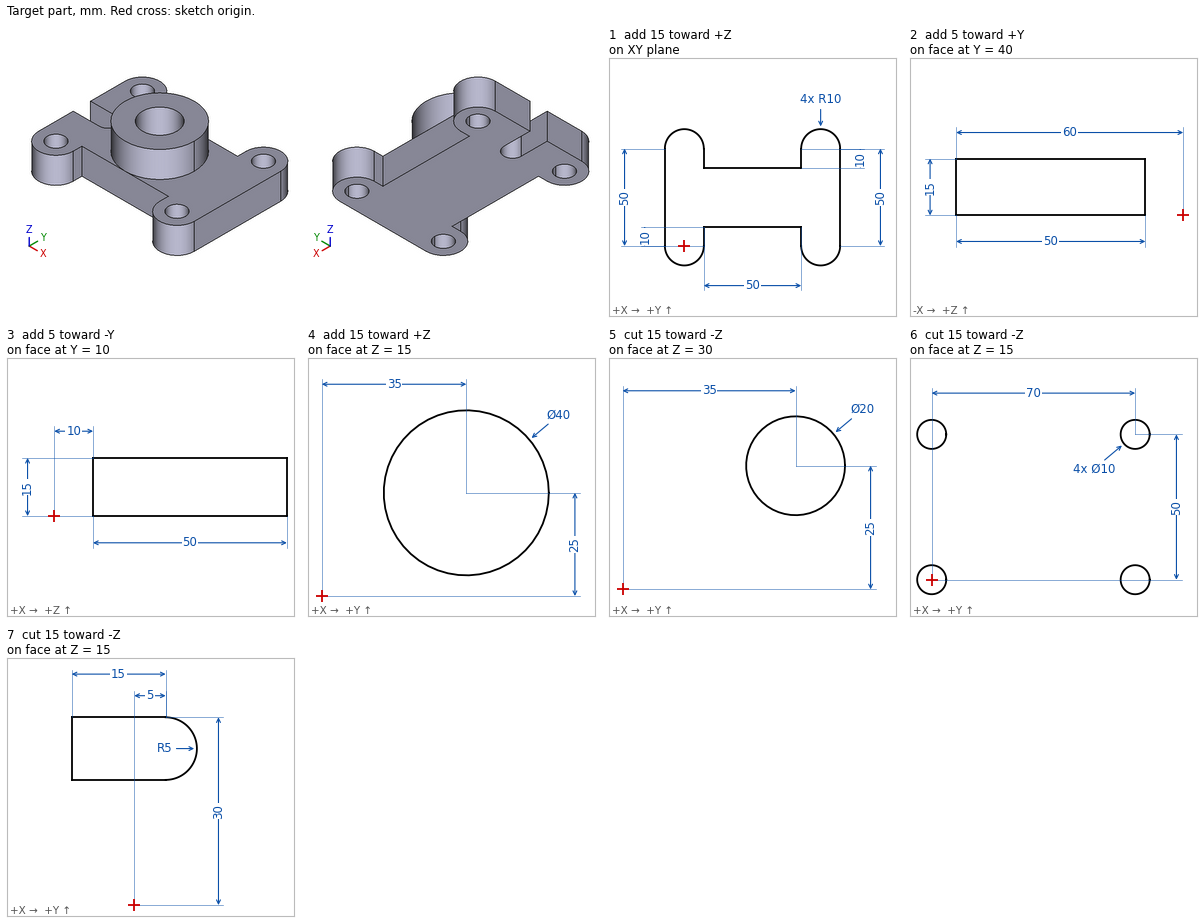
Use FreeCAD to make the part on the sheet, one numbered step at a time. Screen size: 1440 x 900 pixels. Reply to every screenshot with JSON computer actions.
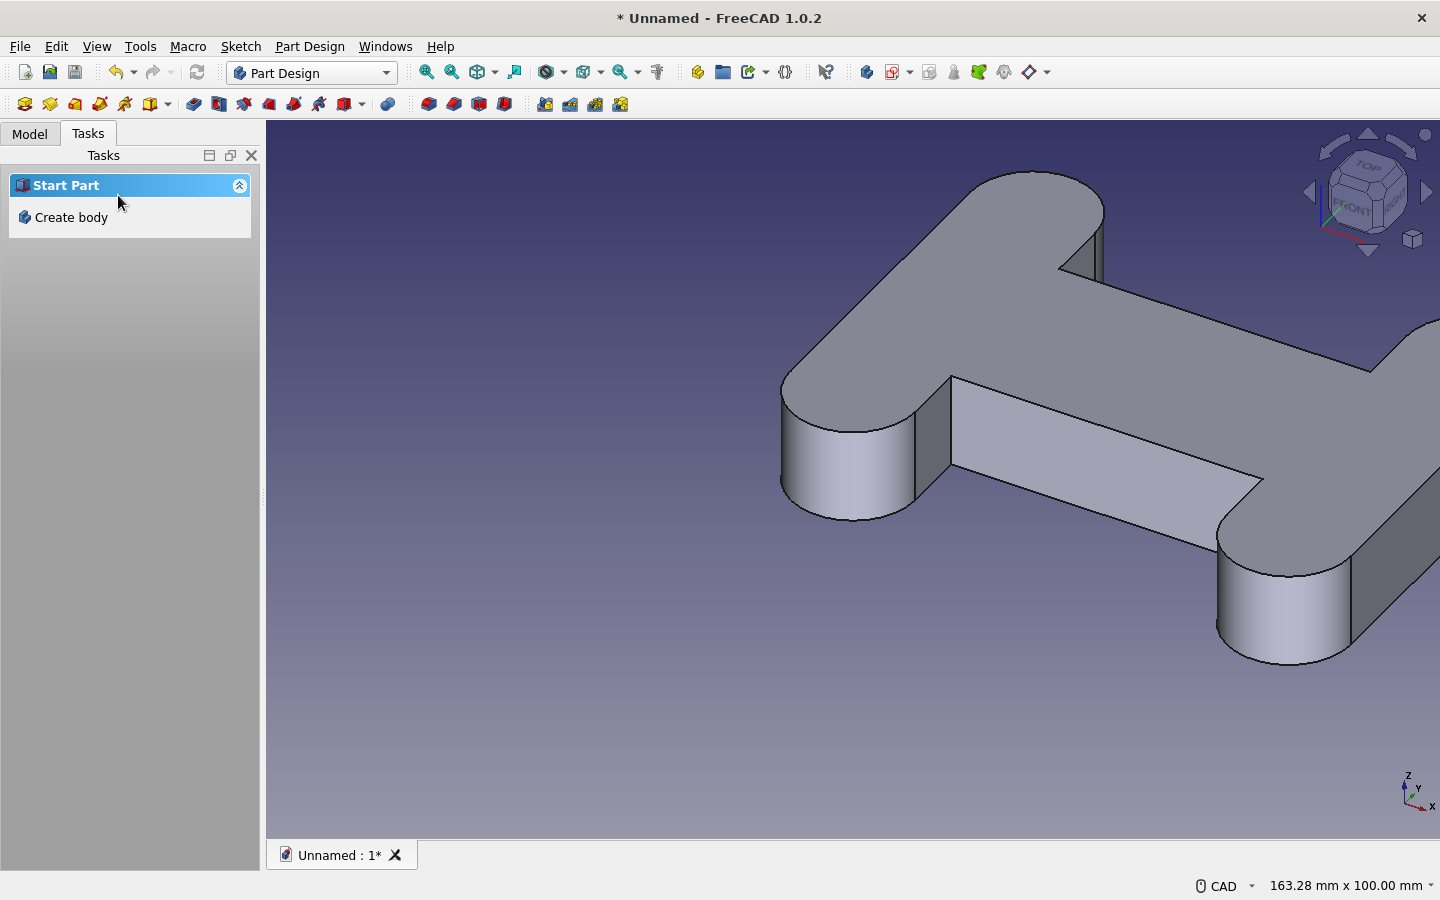
{"action": "left_click", "coordinate": [427, 72]}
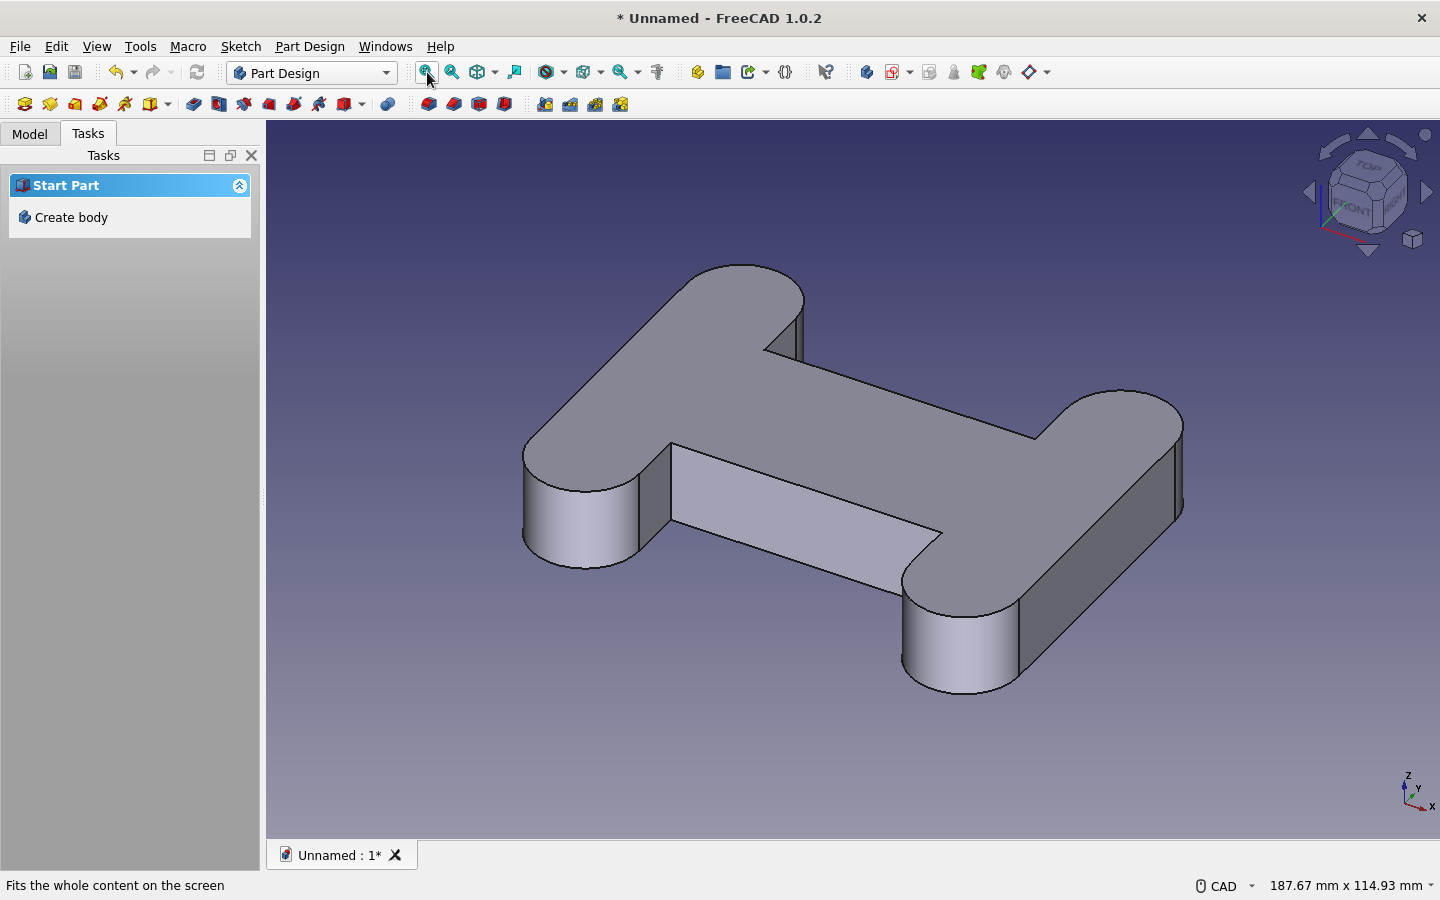
{"action": "key", "text": "4"}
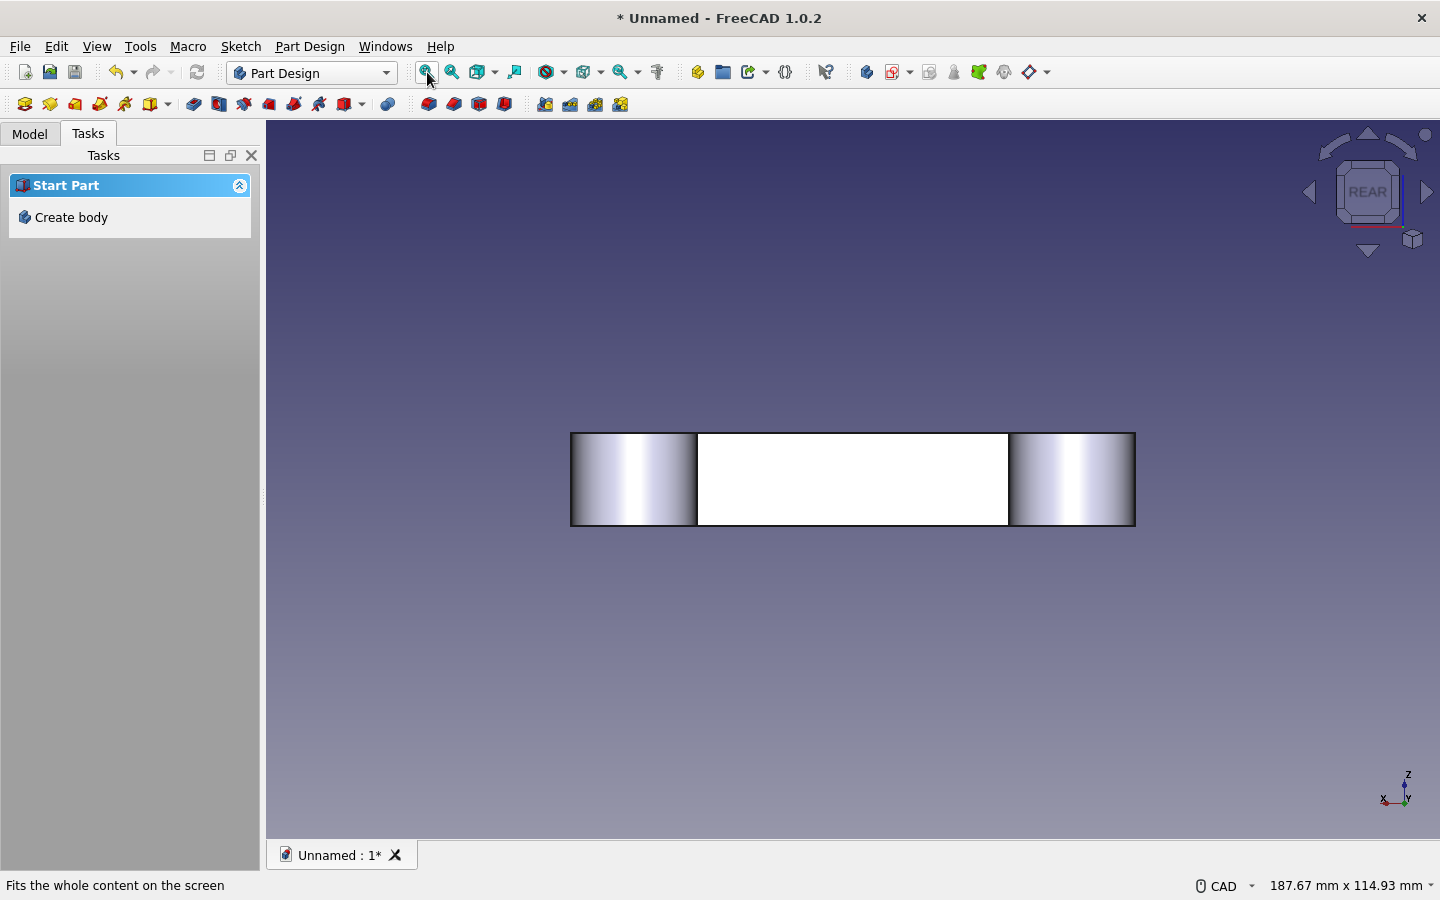
{"action": "left_click", "coordinate": [764, 479]}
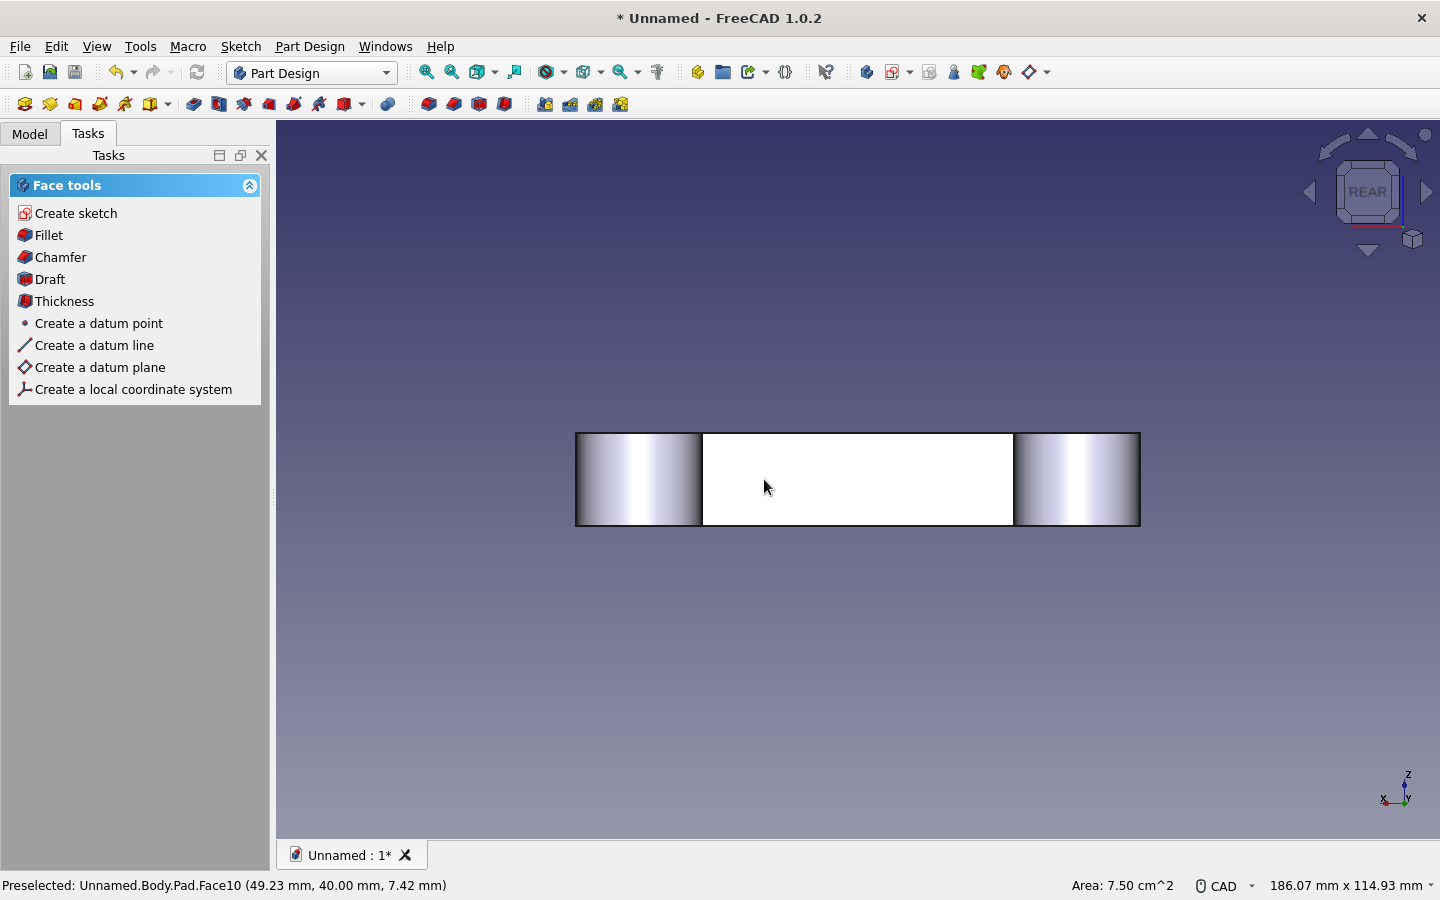
{"action": "left_click", "coordinate": [892, 72]}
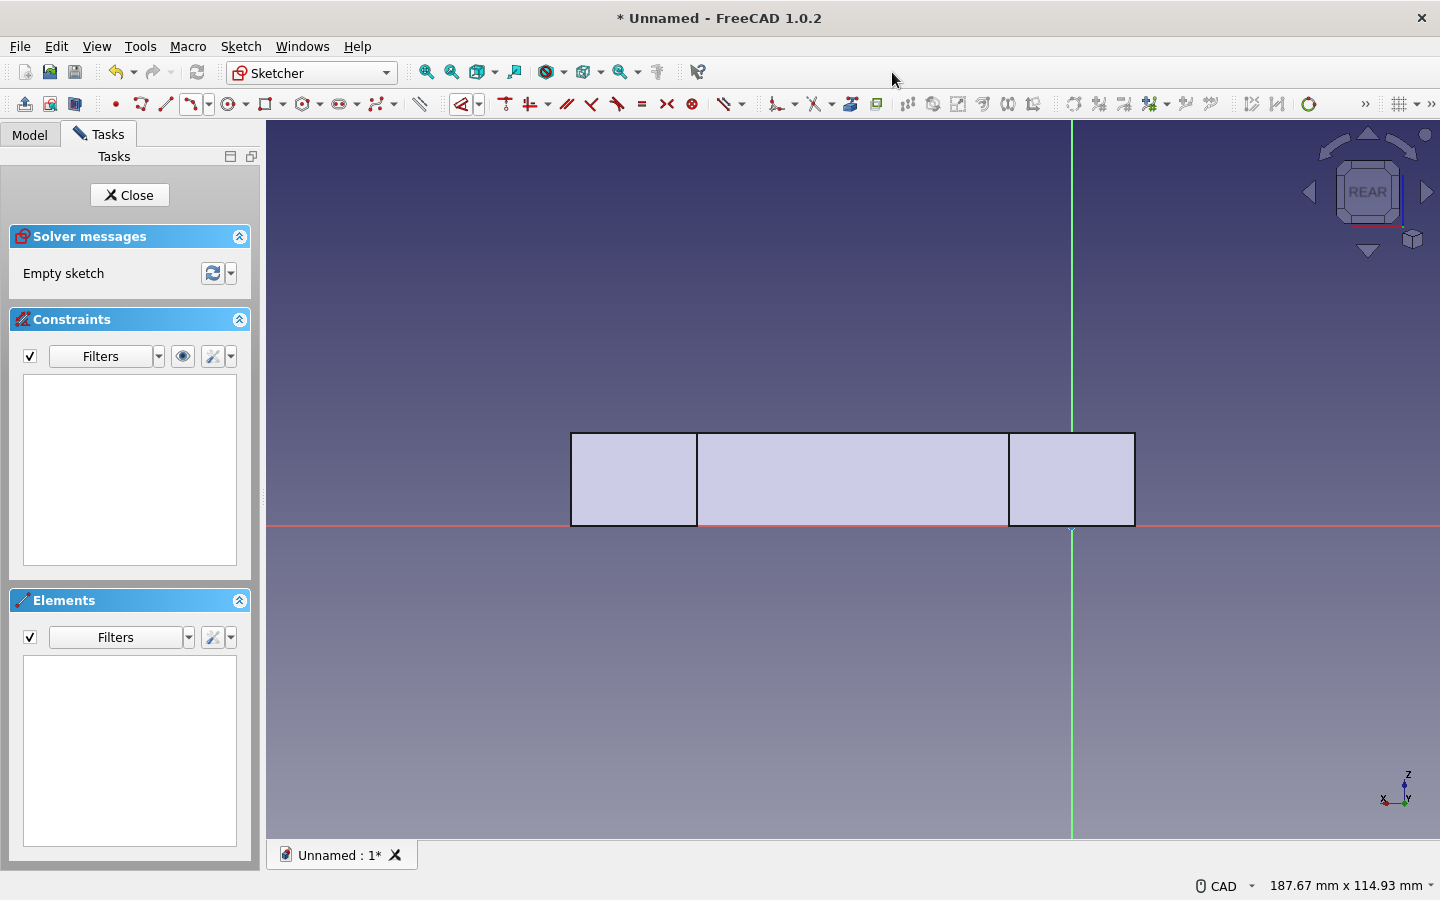
{"action": "left_click", "coordinate": [75, 104]}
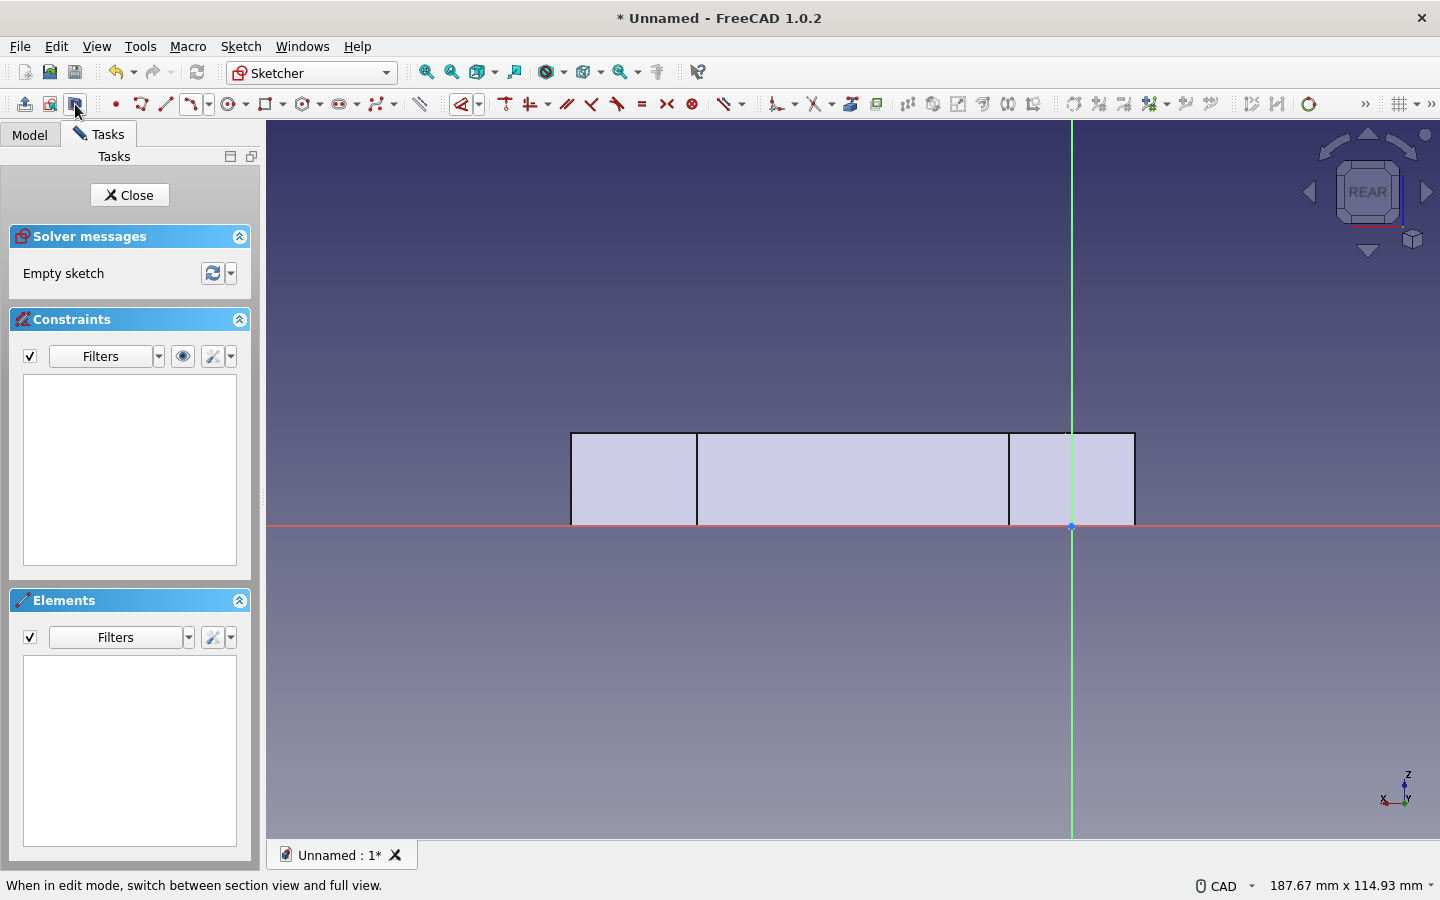
{"action": "scroll", "coordinate": [1006, 480], "scroll_direction": "up", "scroll_amount": 3}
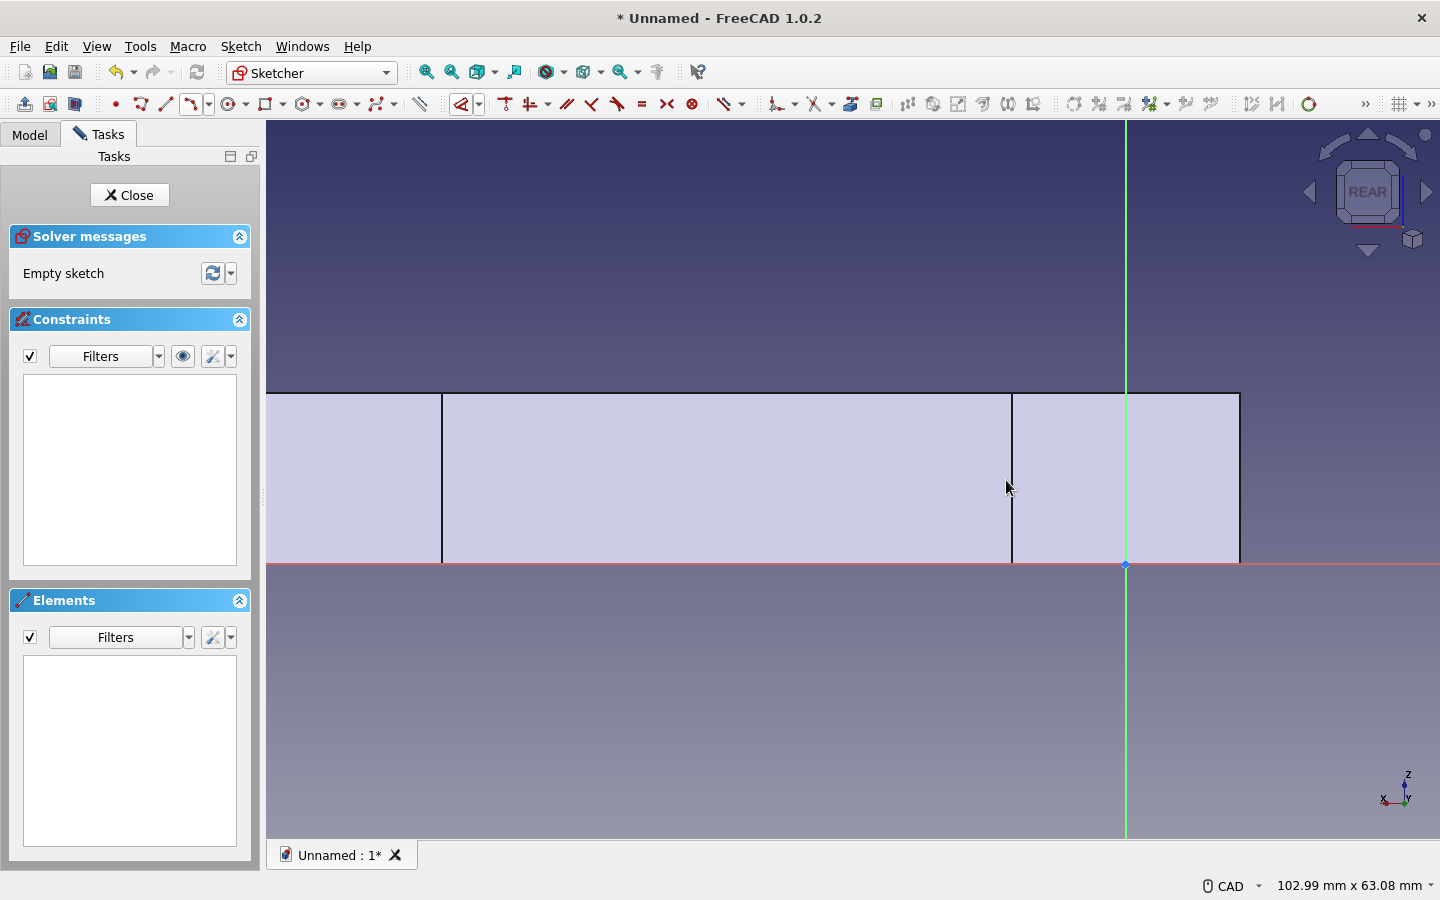
{"action": "left_click", "coordinate": [264, 104]}